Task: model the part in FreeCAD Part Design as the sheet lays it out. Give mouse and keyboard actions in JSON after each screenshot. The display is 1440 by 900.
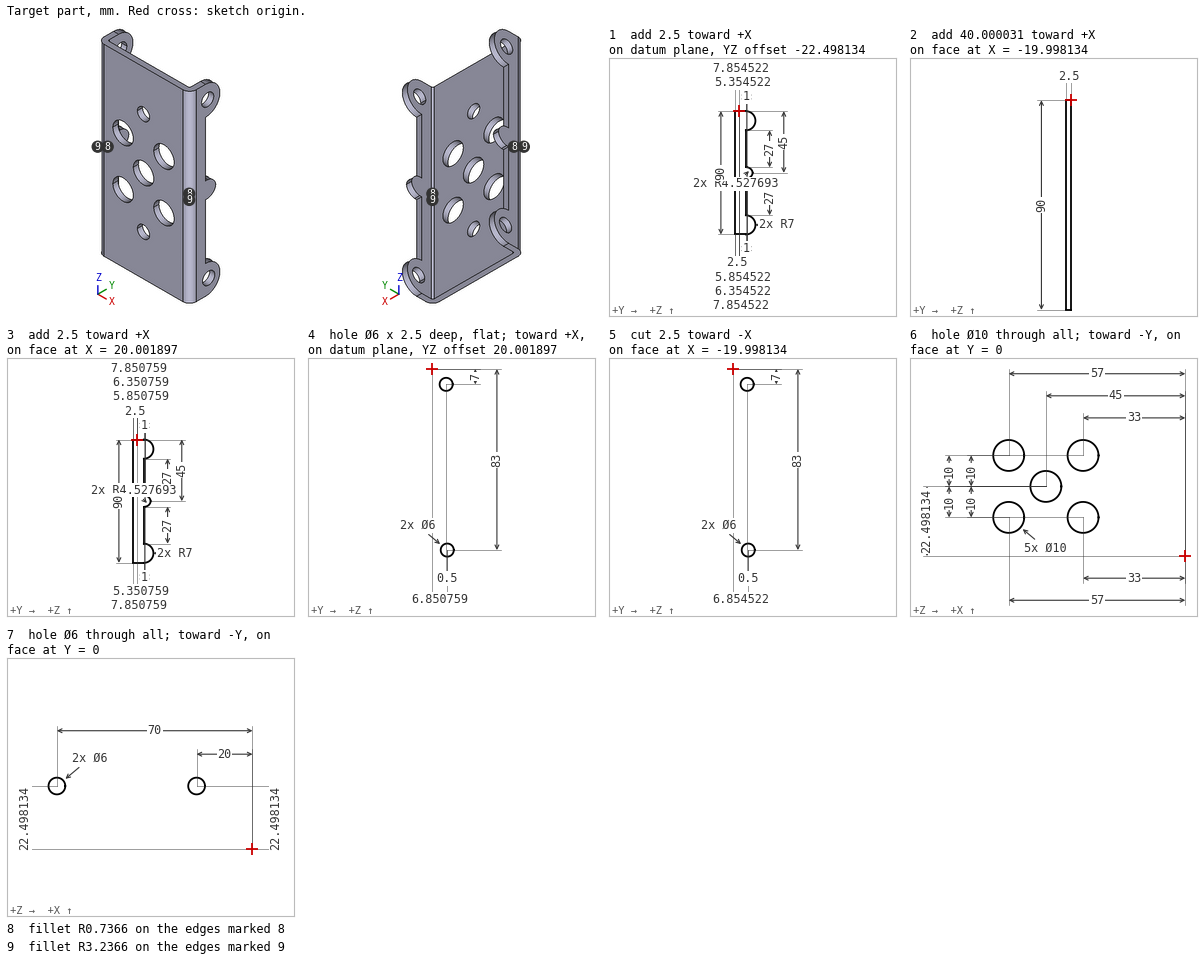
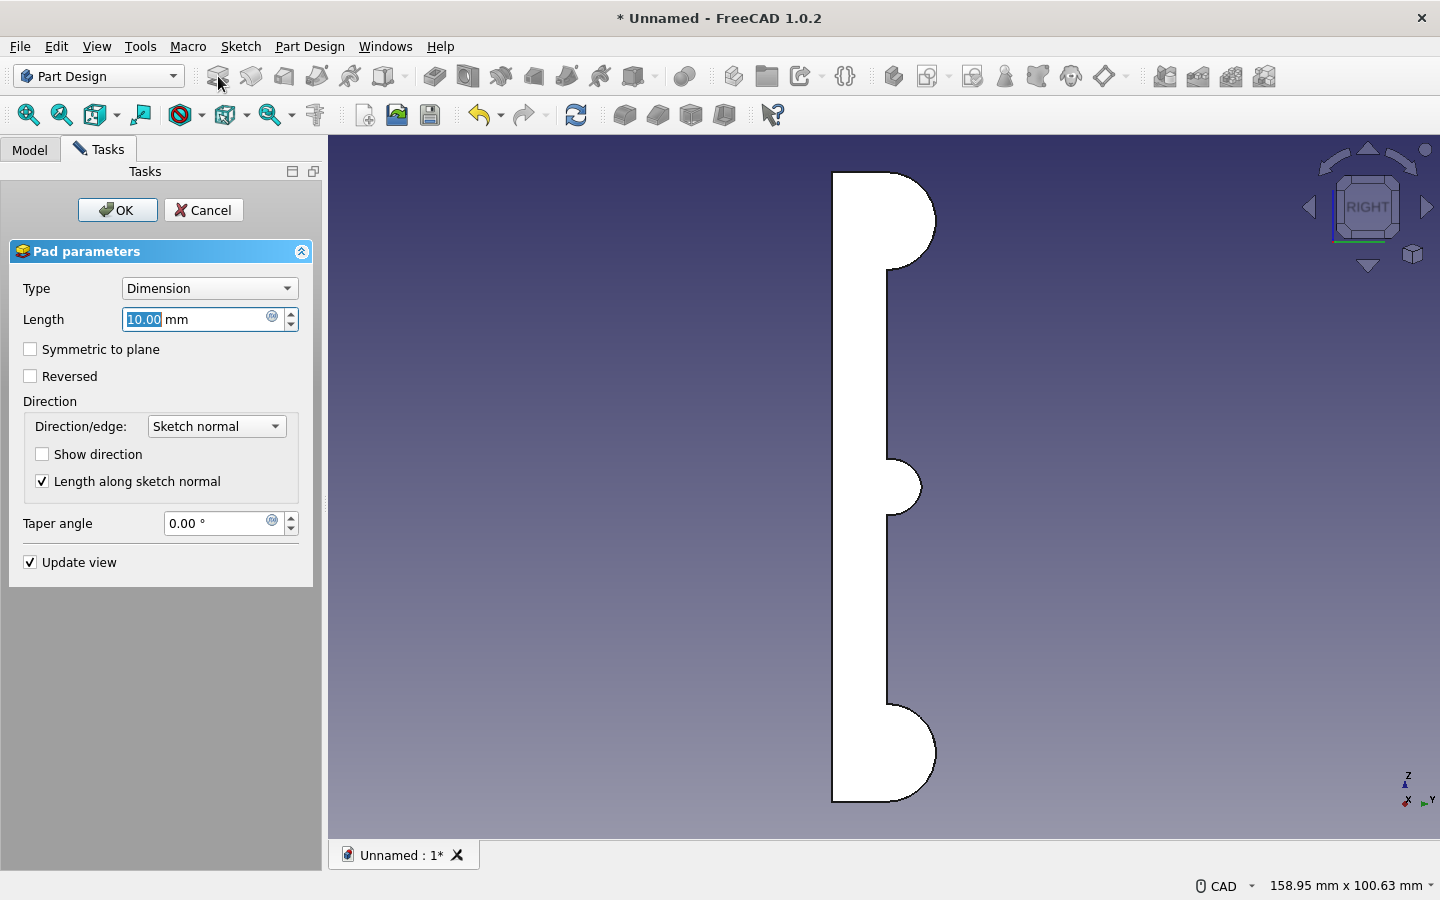
{"action": "type", "text": "2.5"}
{"action": "key", "text": "Tab"}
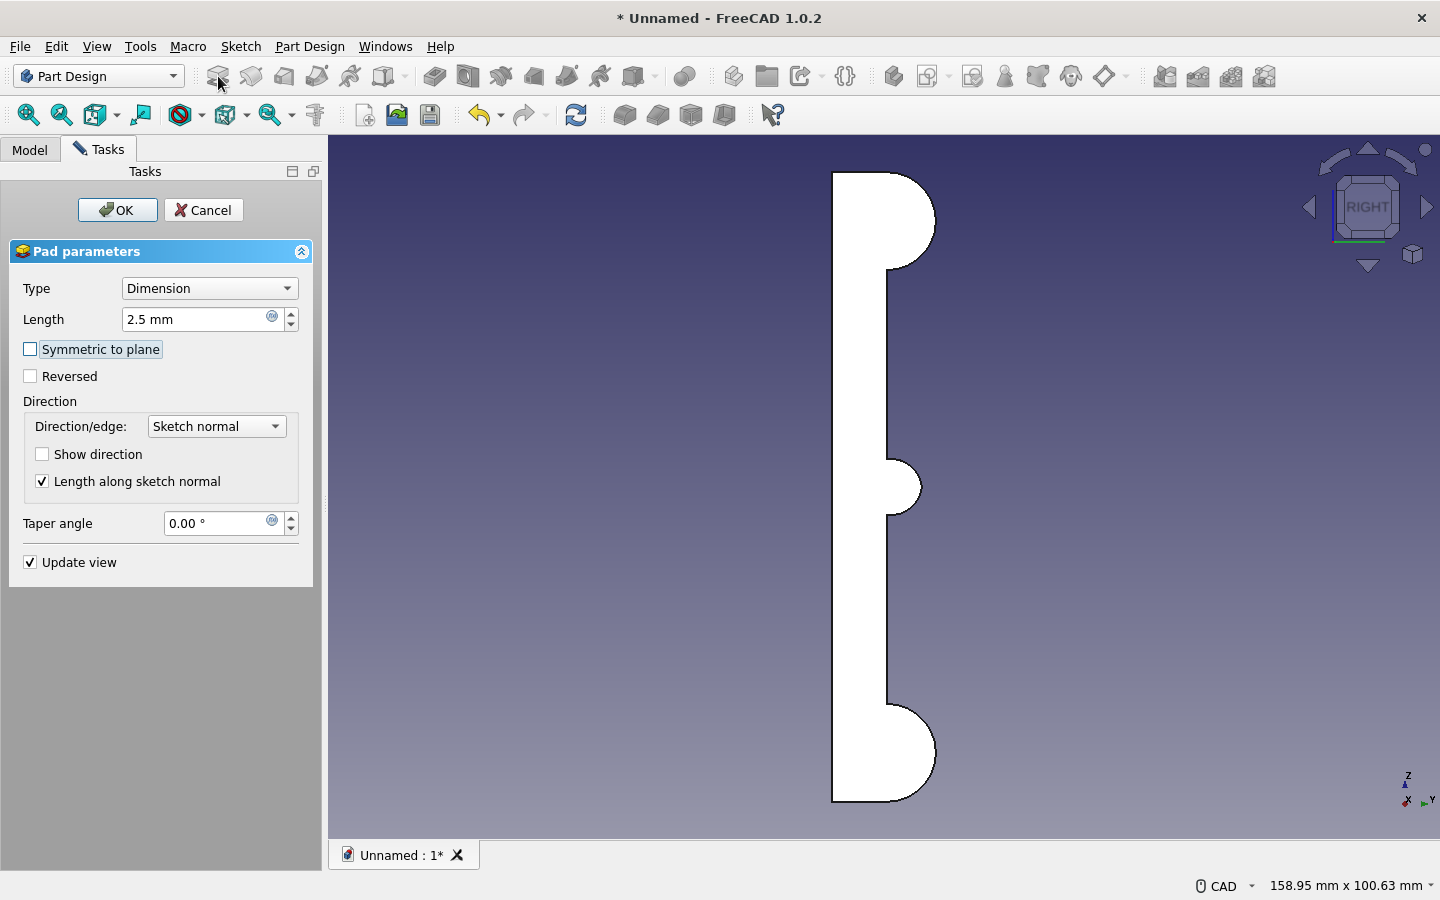
{"action": "left_click", "coordinate": [118, 210]}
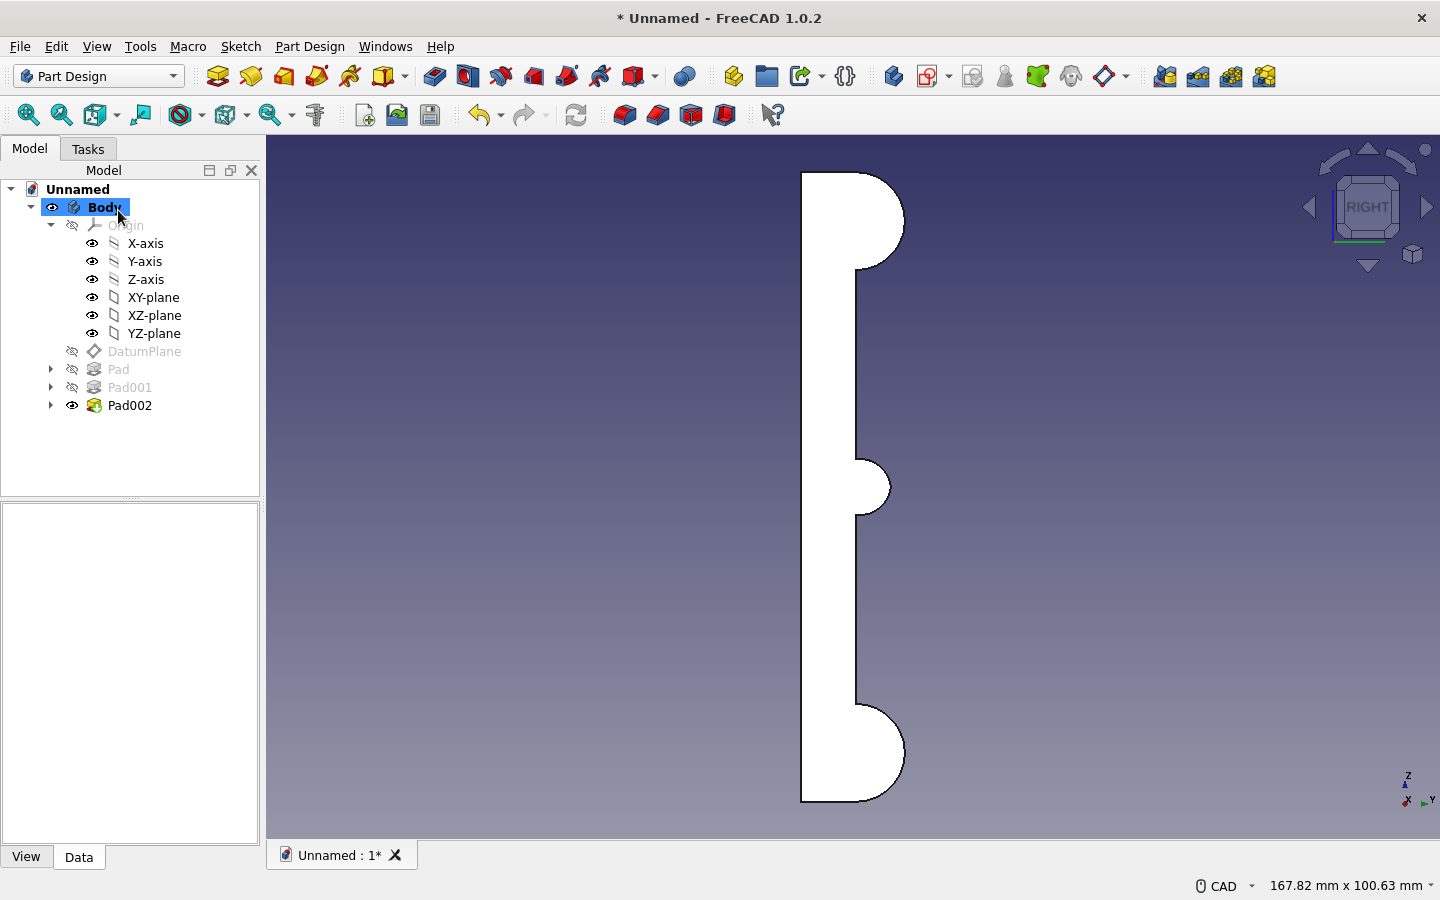
{"action": "left_click", "coordinate": [137, 333]}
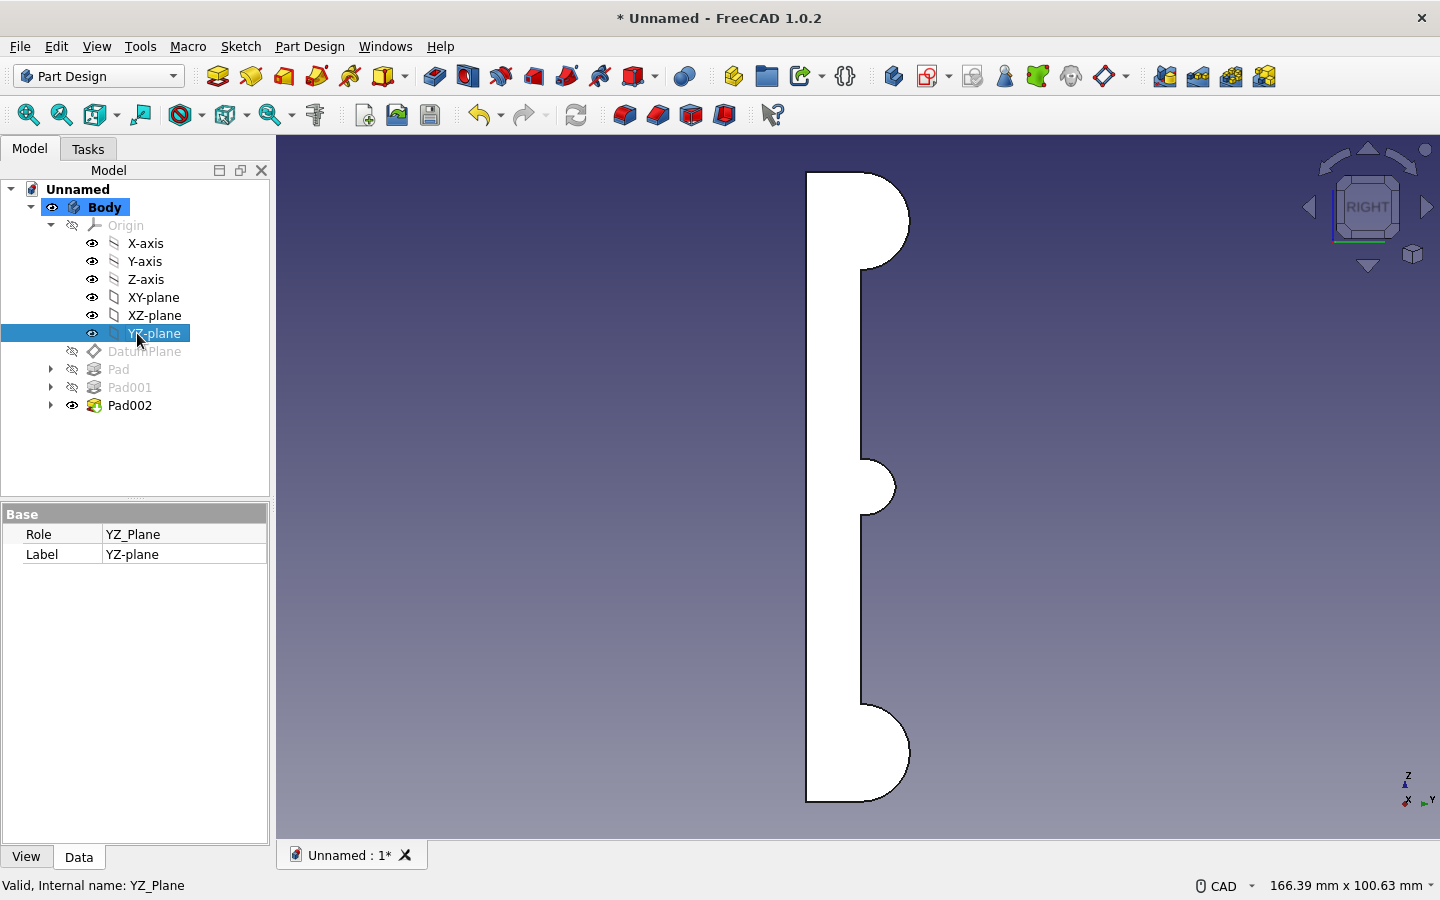
{"action": "left_click", "coordinate": [1104, 76]}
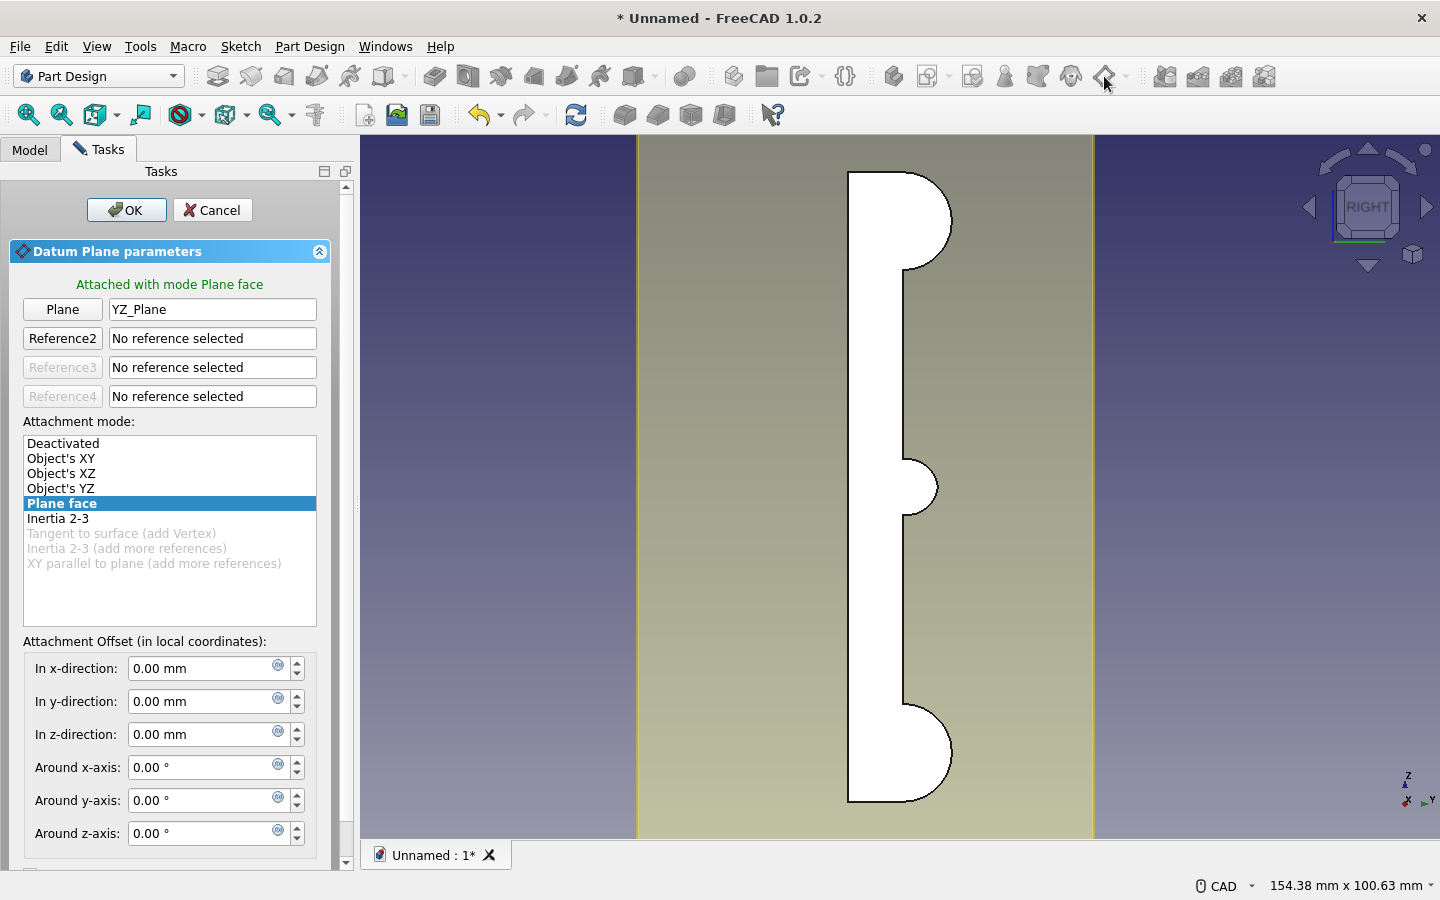
{"action": "triple_click", "coordinate": [210, 734]}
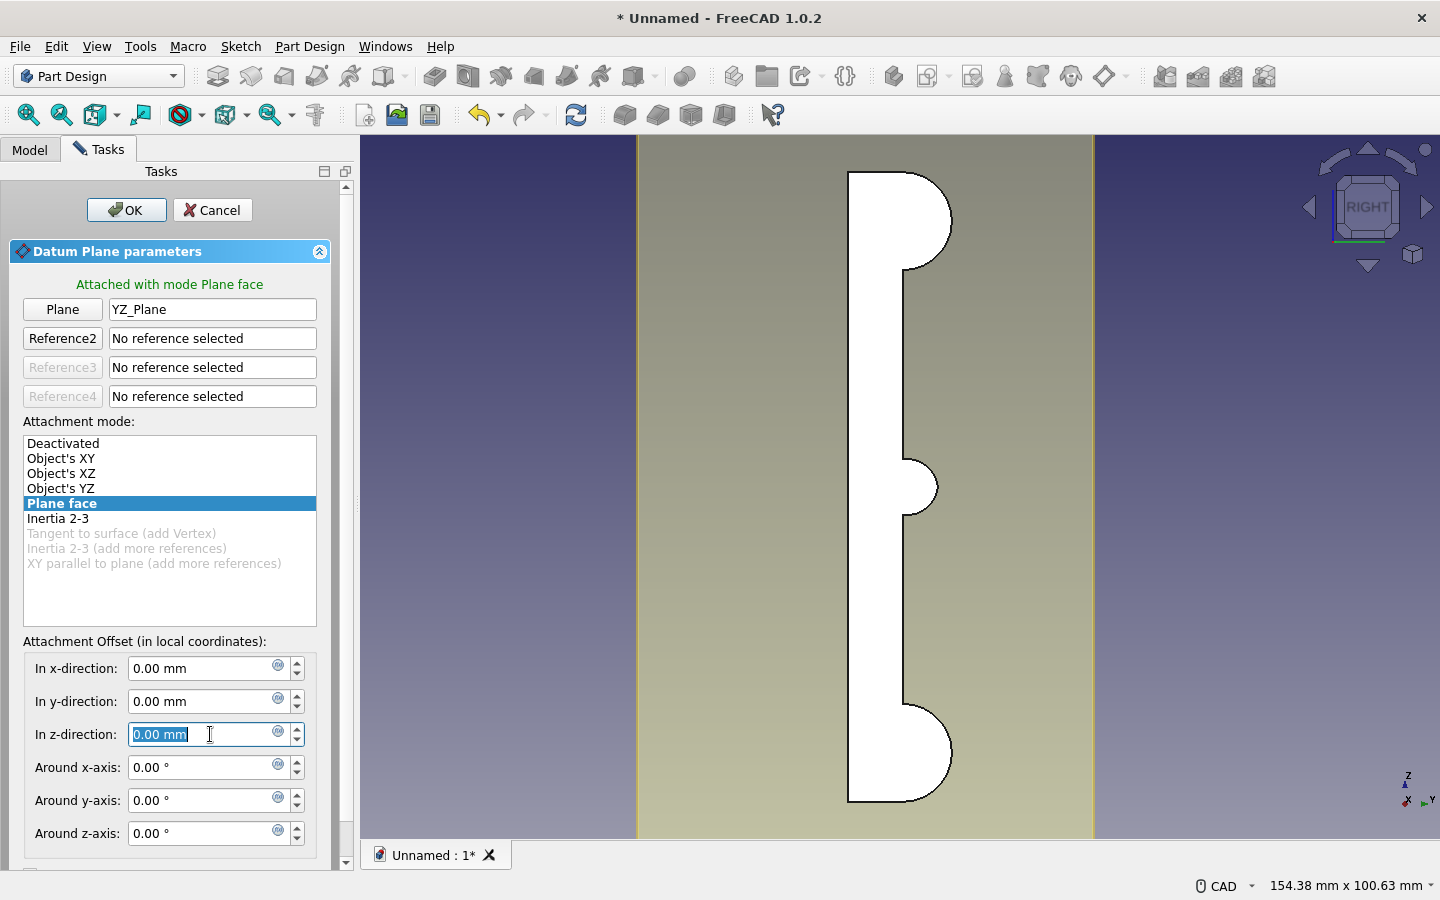
{"action": "type", "text": "20.001897"}
{"action": "key", "text": "Tab"}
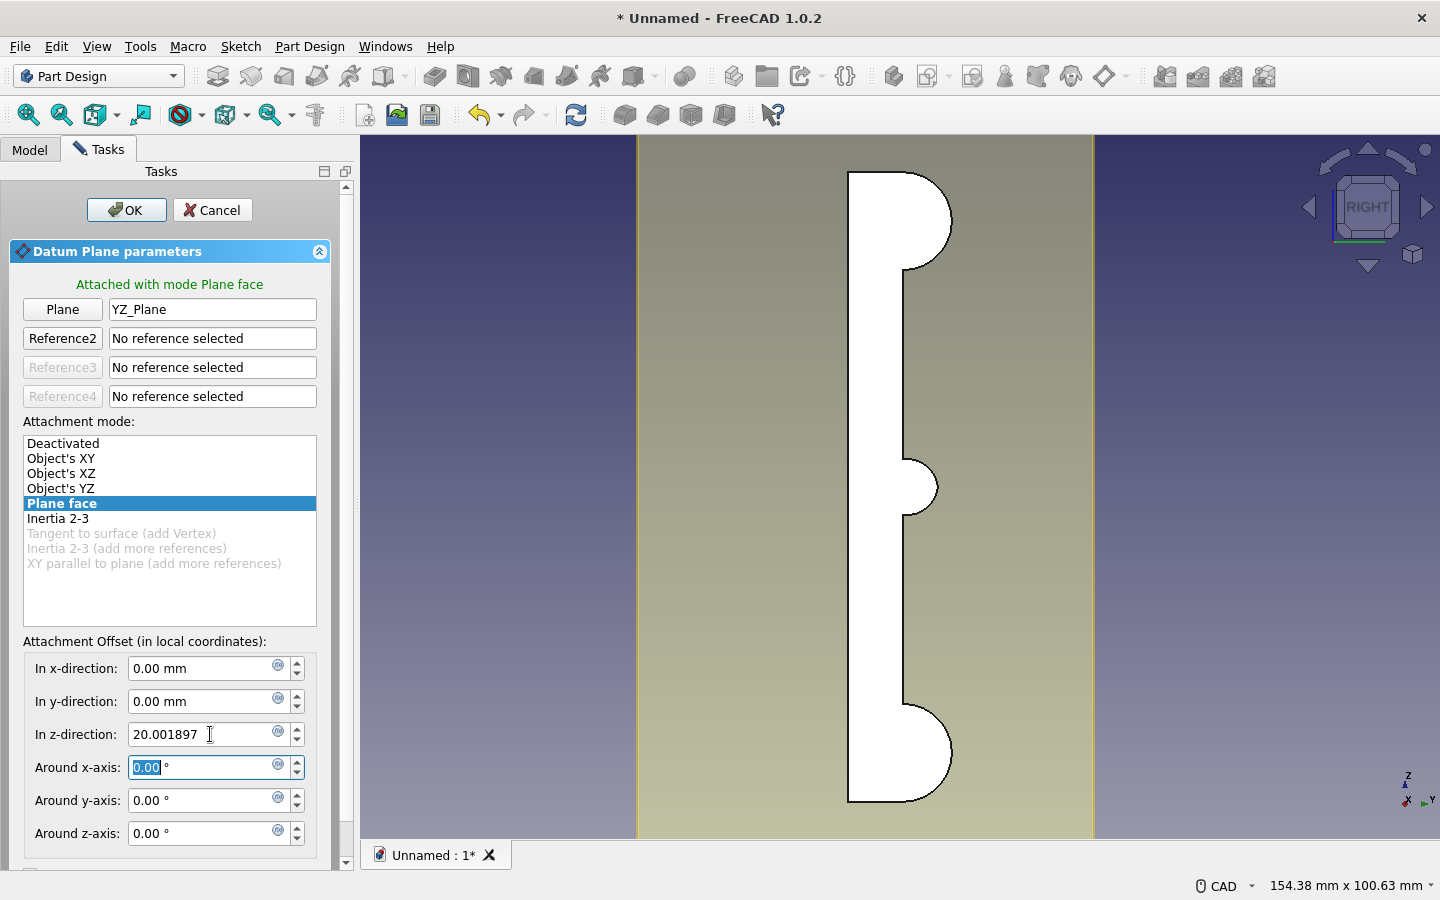
{"action": "left_click", "coordinate": [127, 210]}